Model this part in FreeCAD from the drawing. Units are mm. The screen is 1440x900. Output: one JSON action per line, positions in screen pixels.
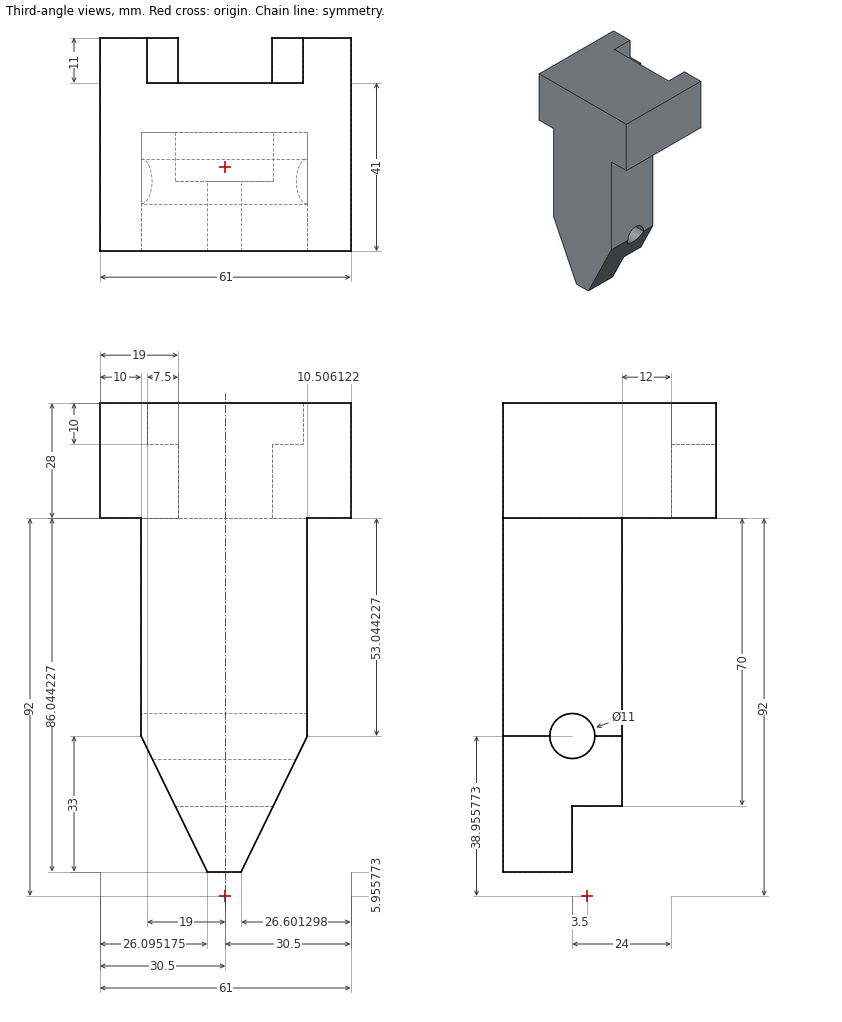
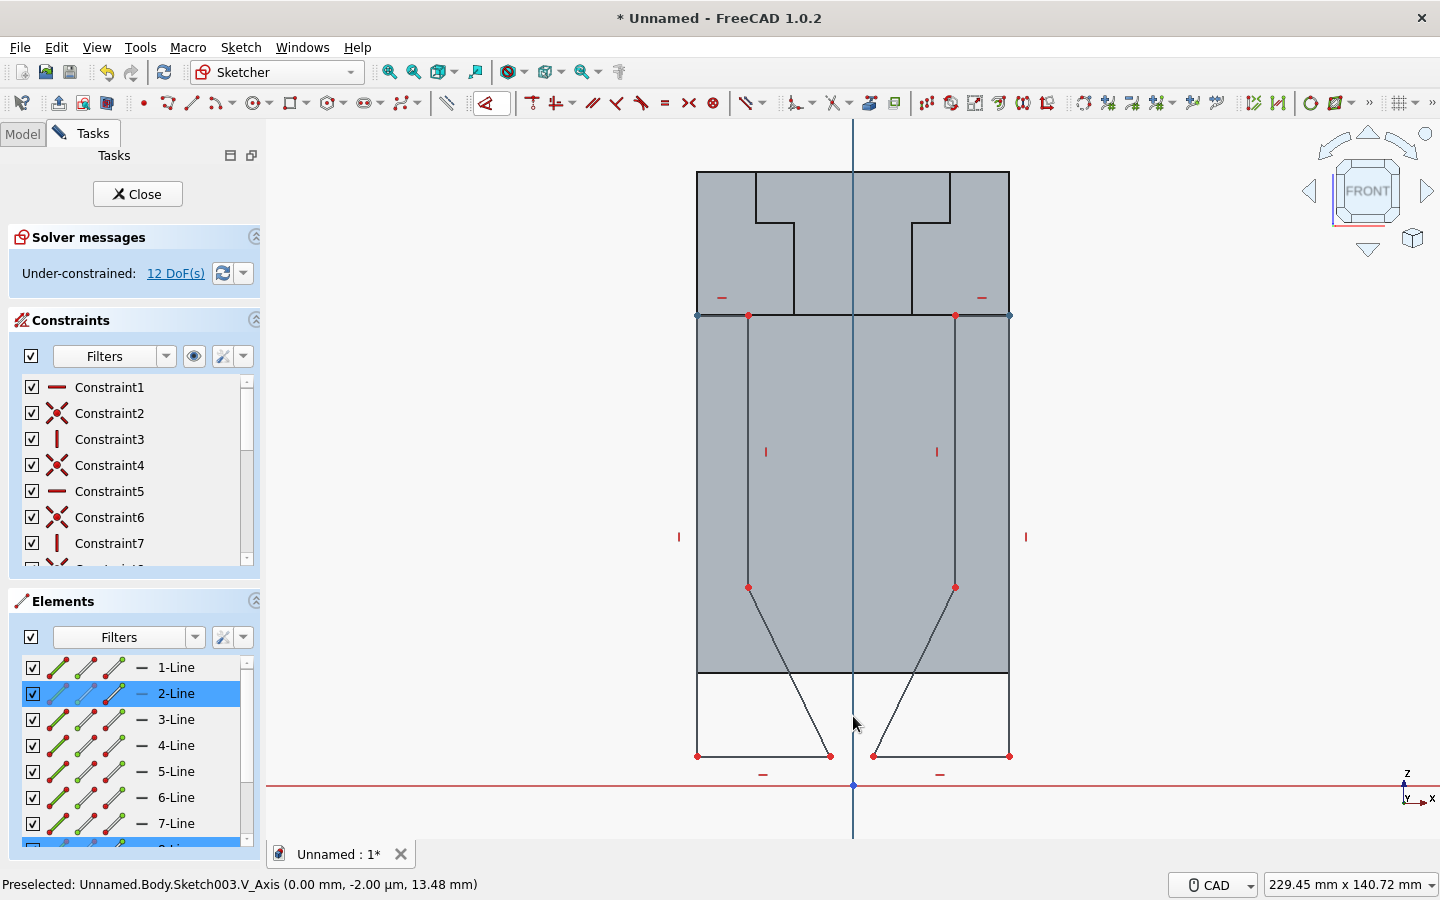
{"action": "left_click", "coordinate": [690, 104]}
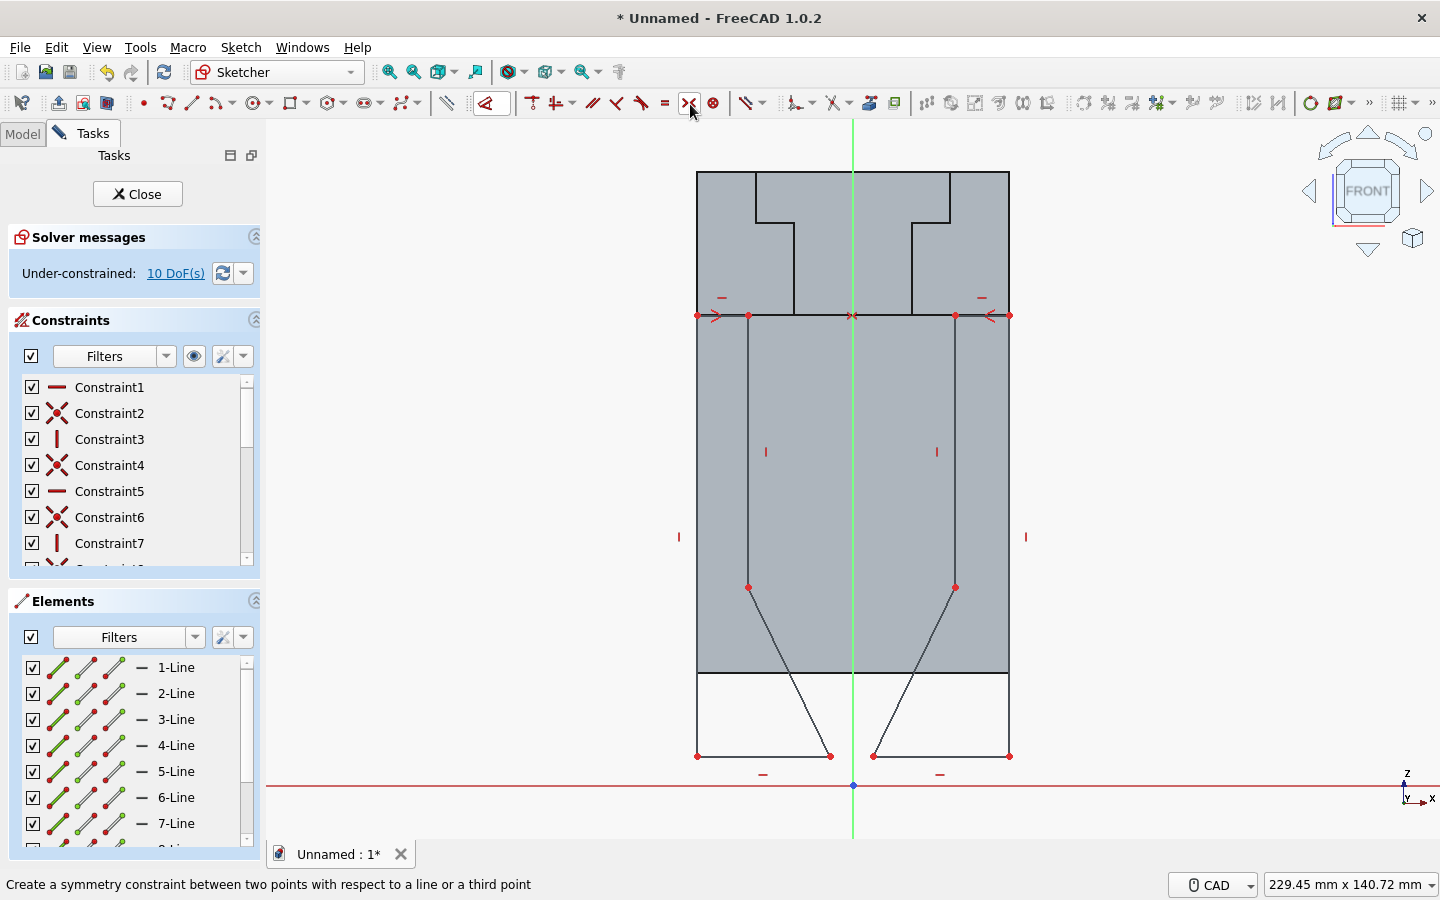
{"action": "left_click", "coordinate": [712, 316]}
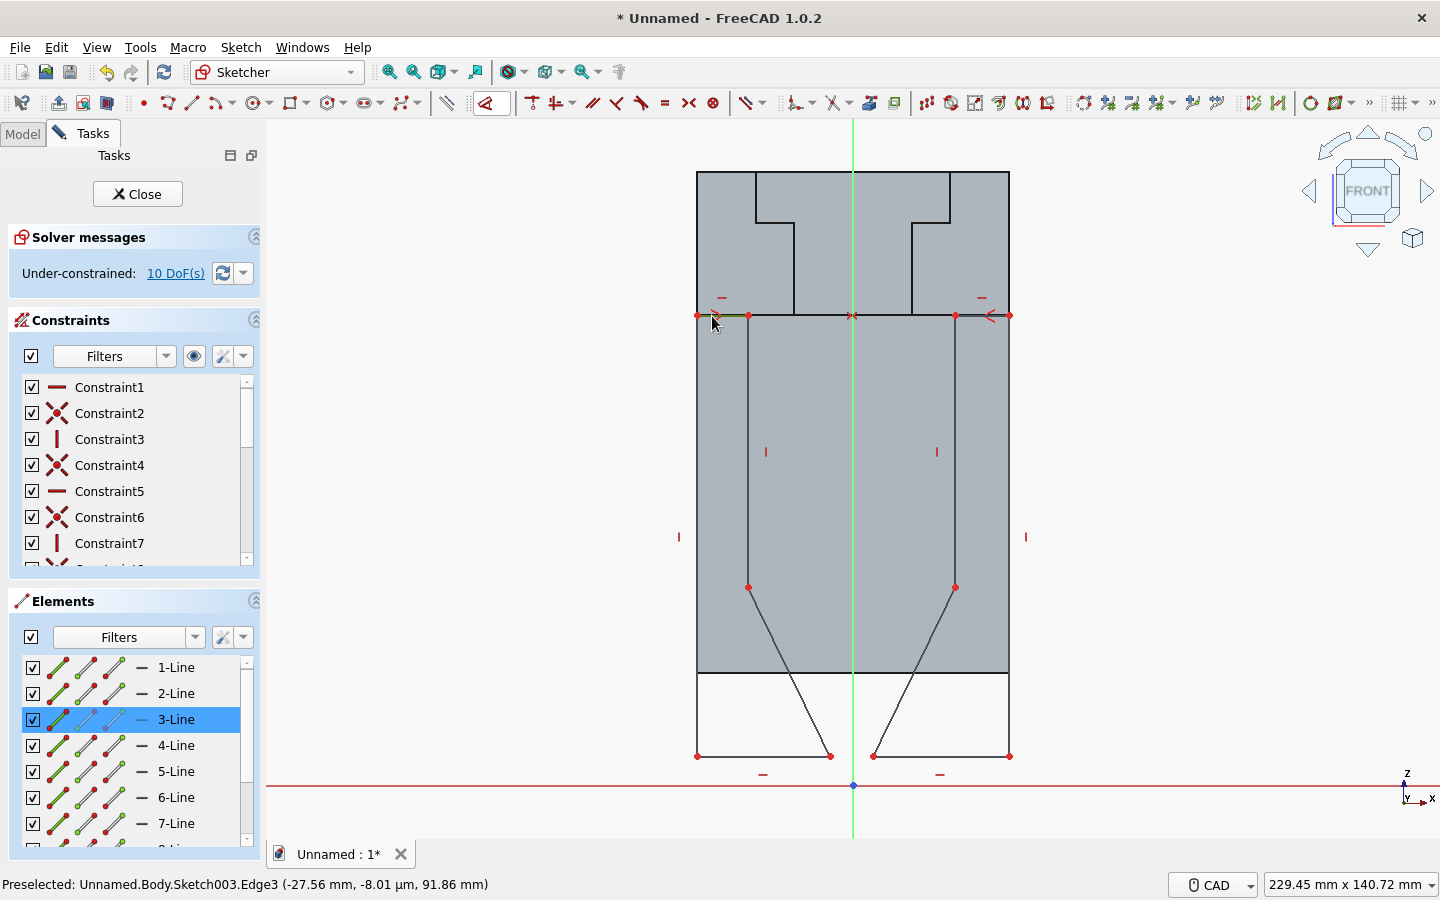
{"action": "left_click", "coordinate": [504, 104]}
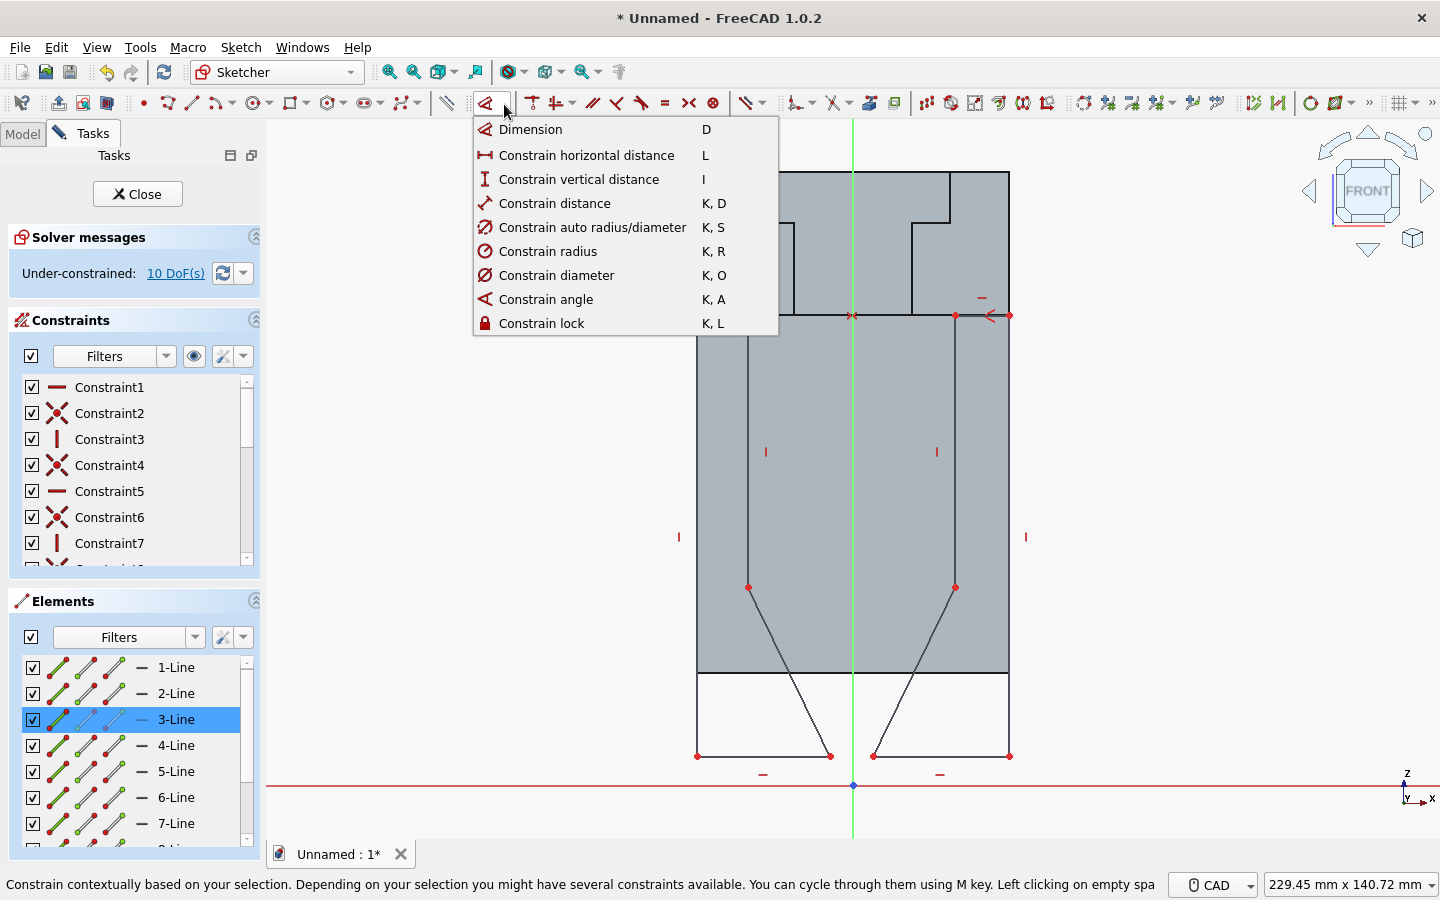
{"action": "left_click", "coordinate": [626, 155]}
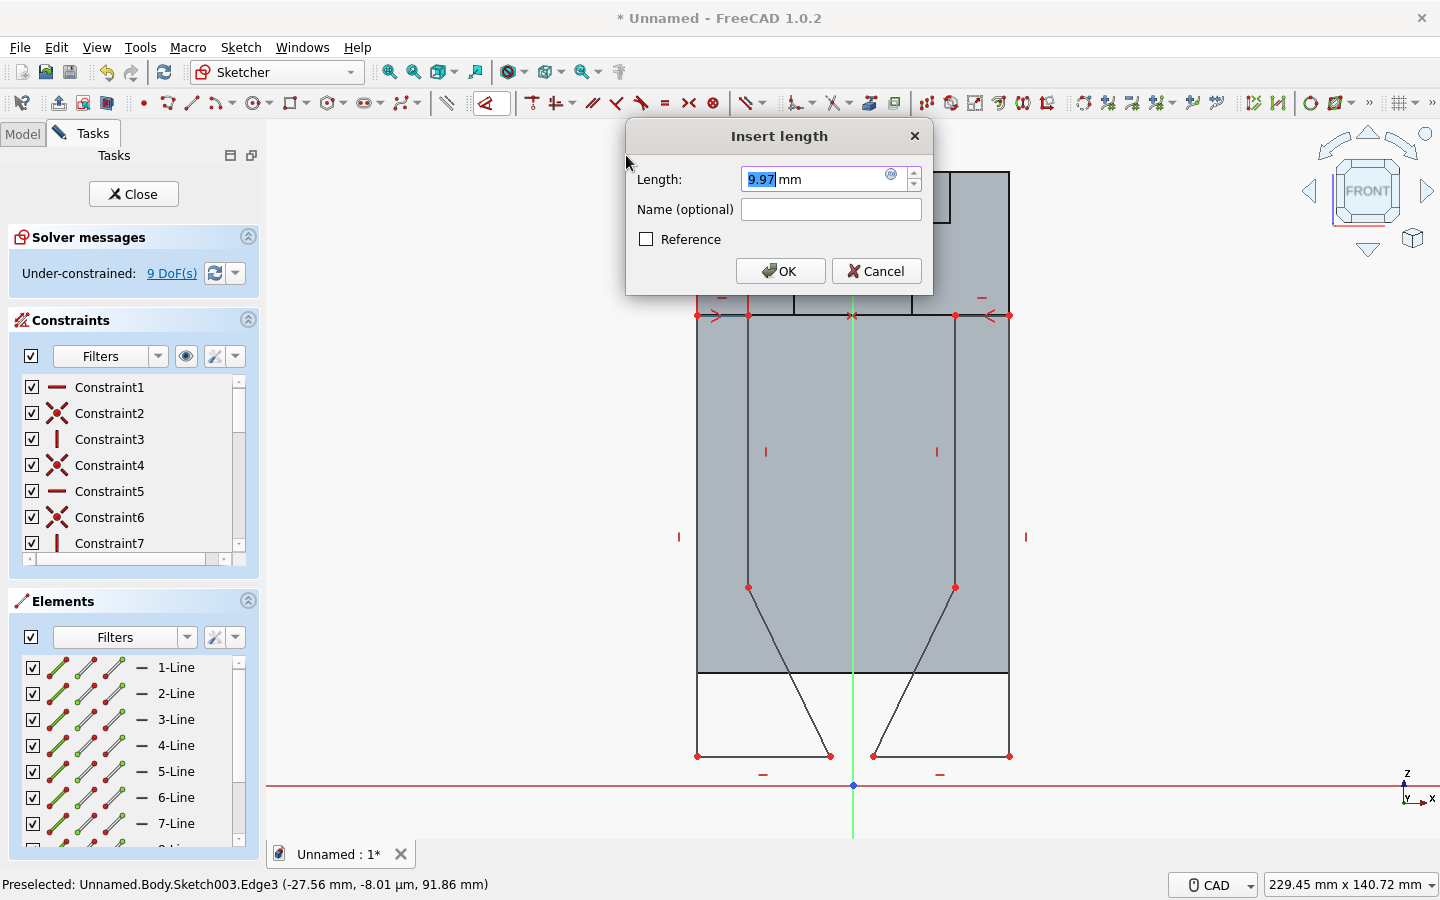
{"action": "type", "text": "10"}
{"action": "key", "text": "Return"}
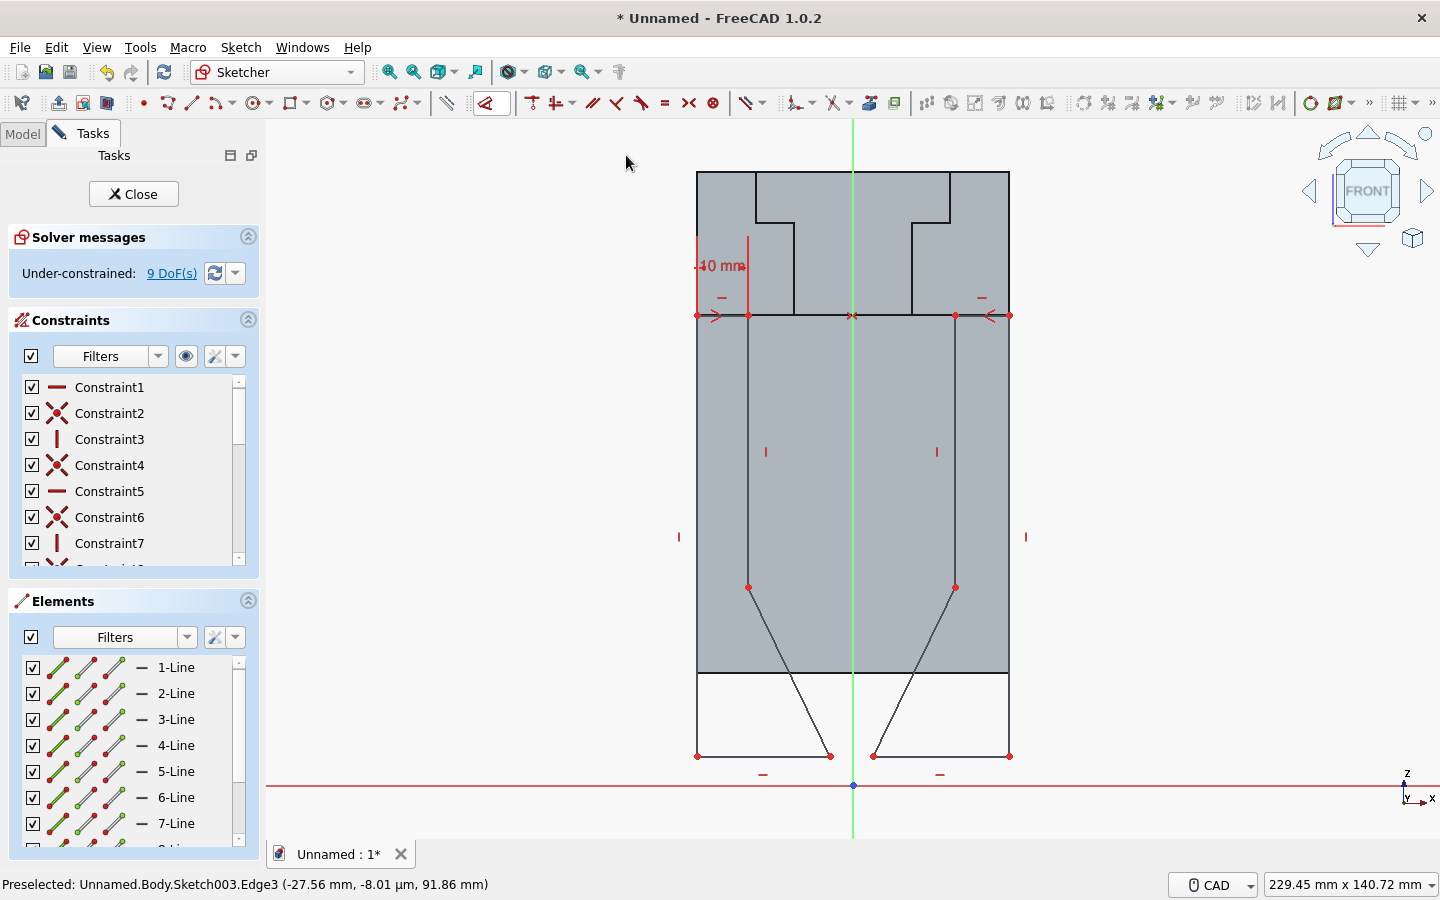
{"action": "left_click", "coordinate": [697, 316]}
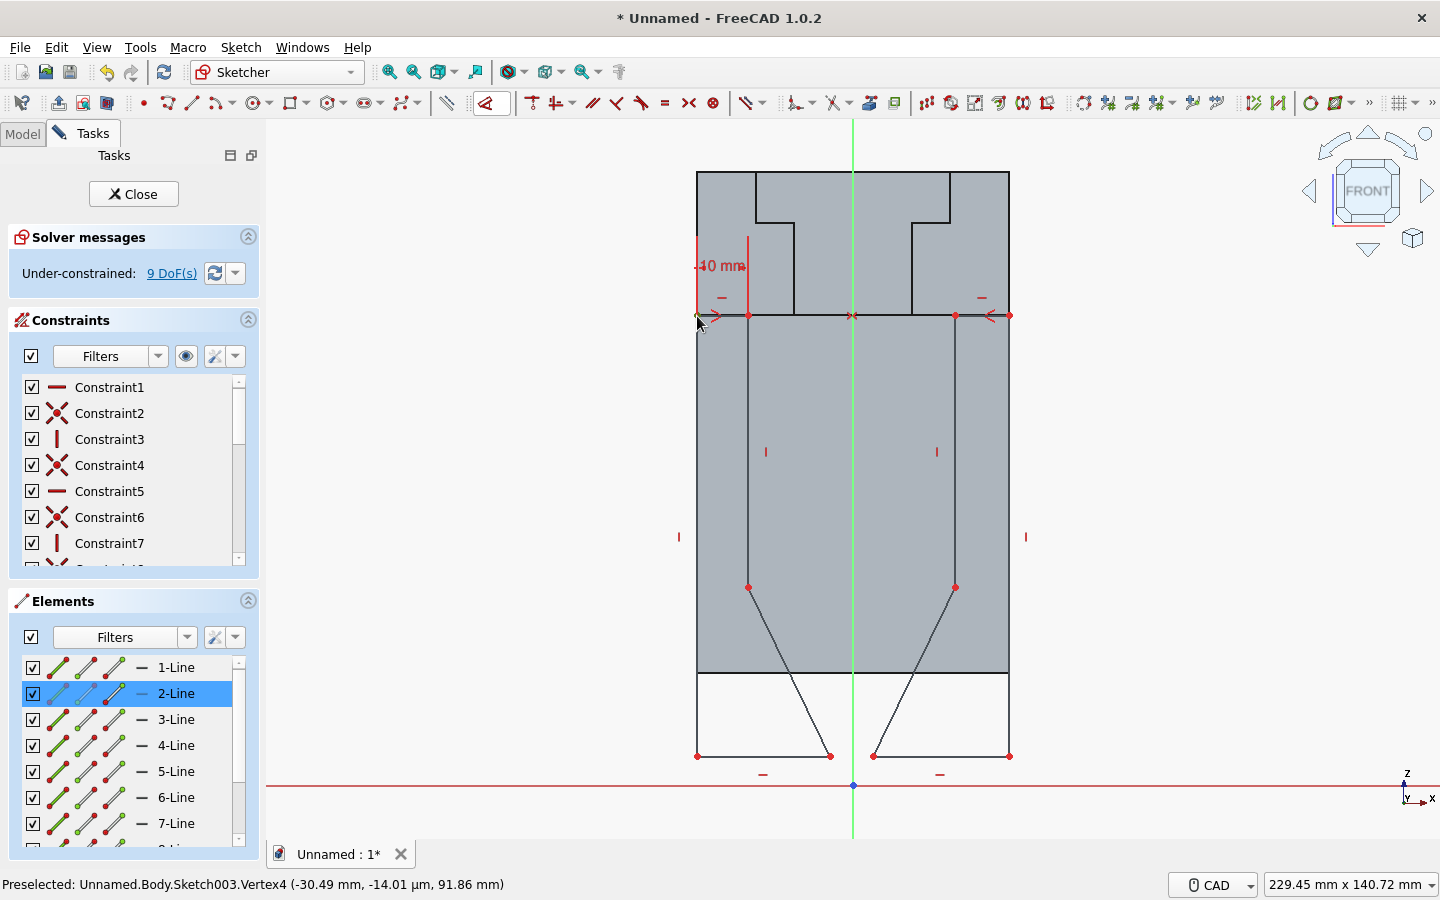
{"action": "left_click", "coordinate": [504, 104]}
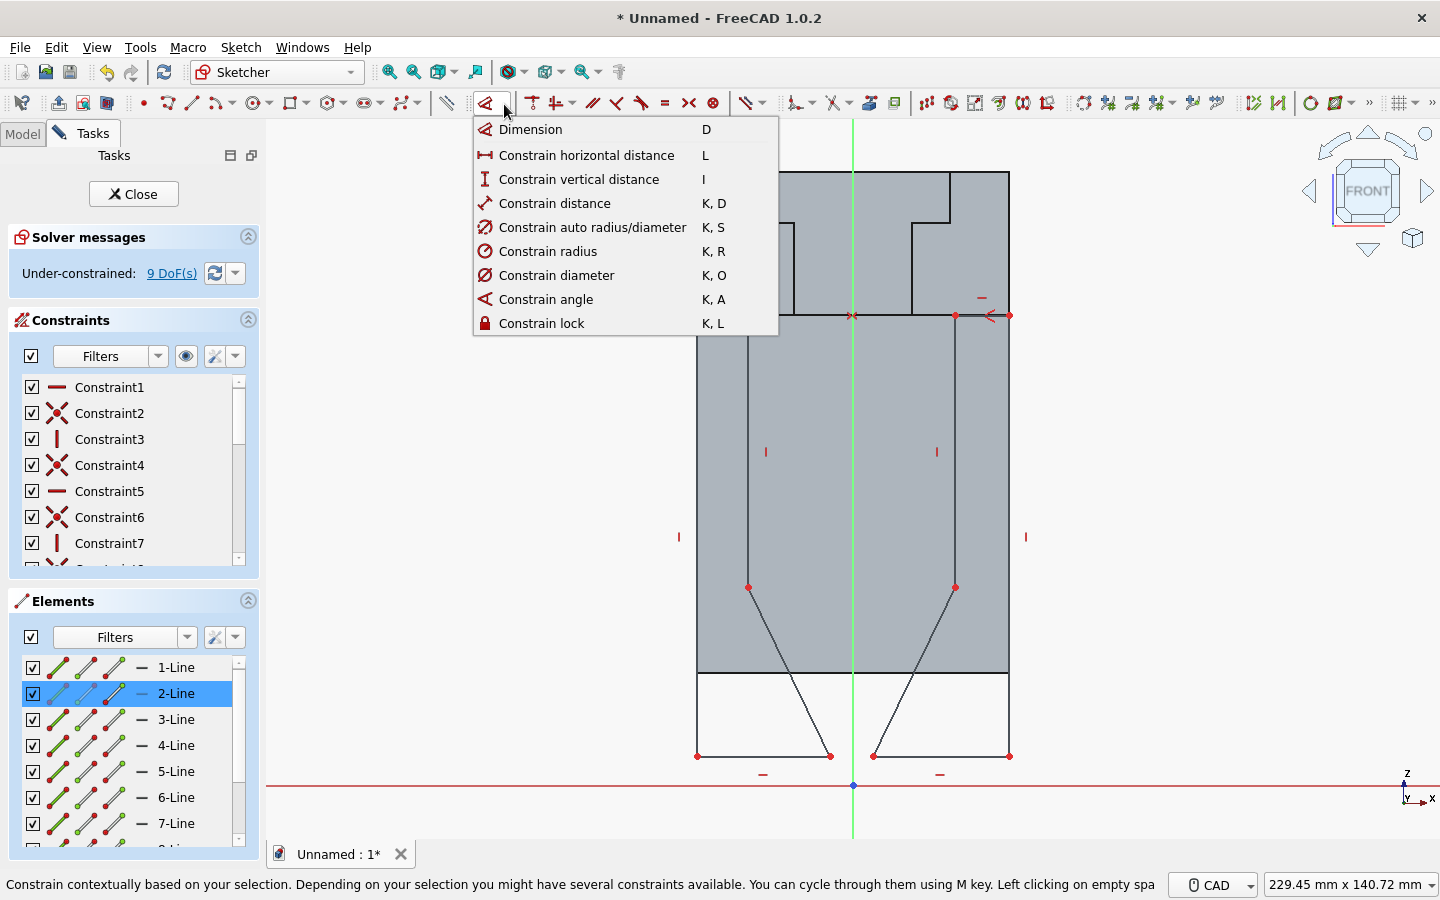
{"action": "left_click", "coordinate": [626, 179]}